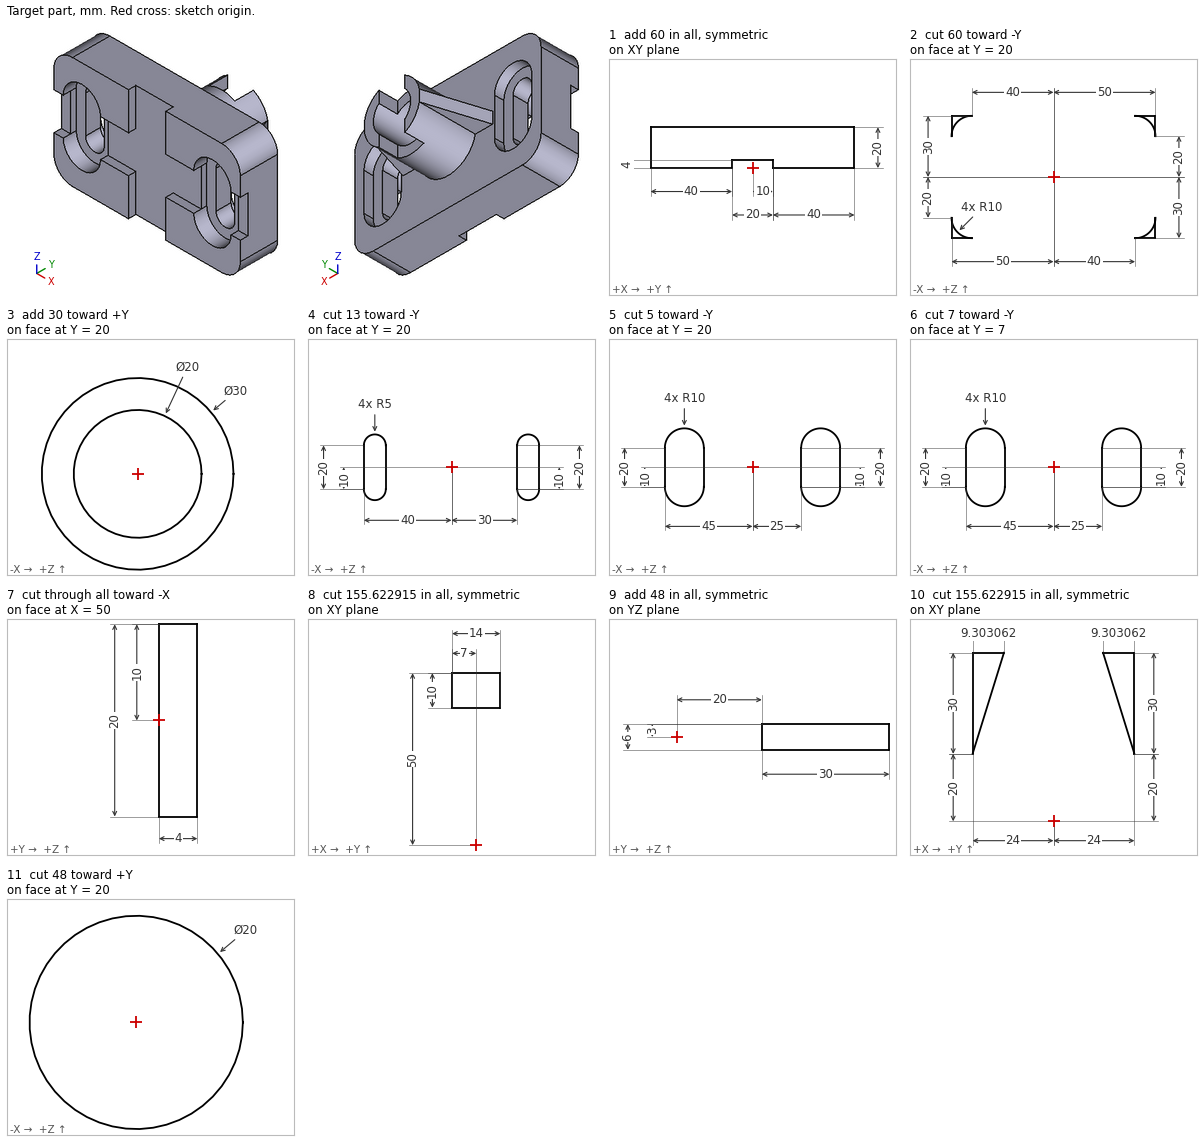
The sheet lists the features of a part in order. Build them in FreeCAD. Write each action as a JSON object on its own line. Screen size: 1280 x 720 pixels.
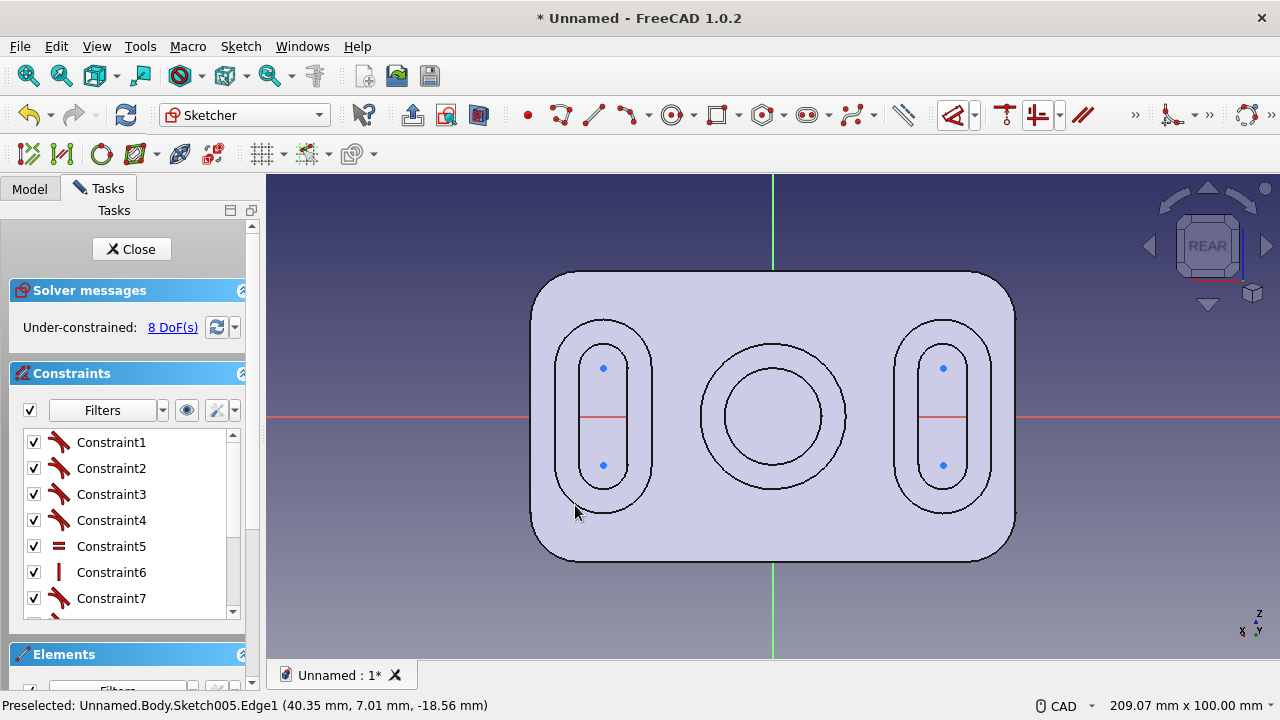
{"action": "left_click", "coordinate": [915, 505]}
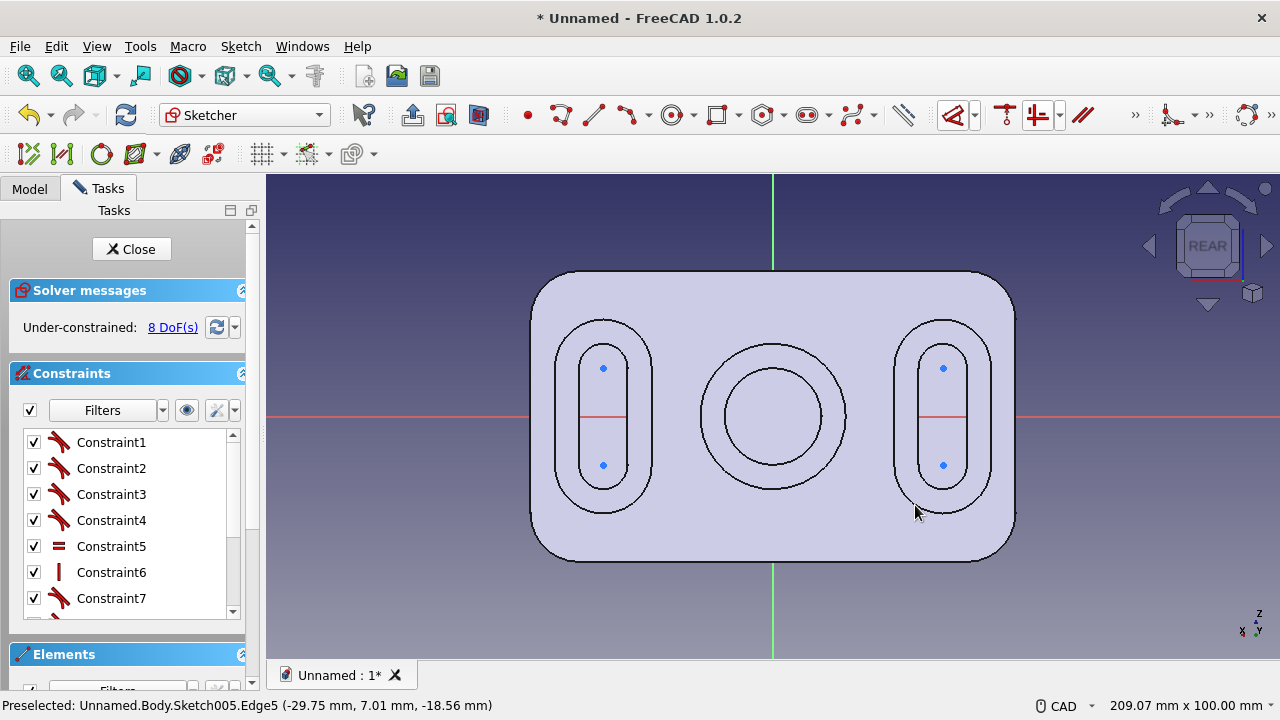
{"action": "key", "text": "e"}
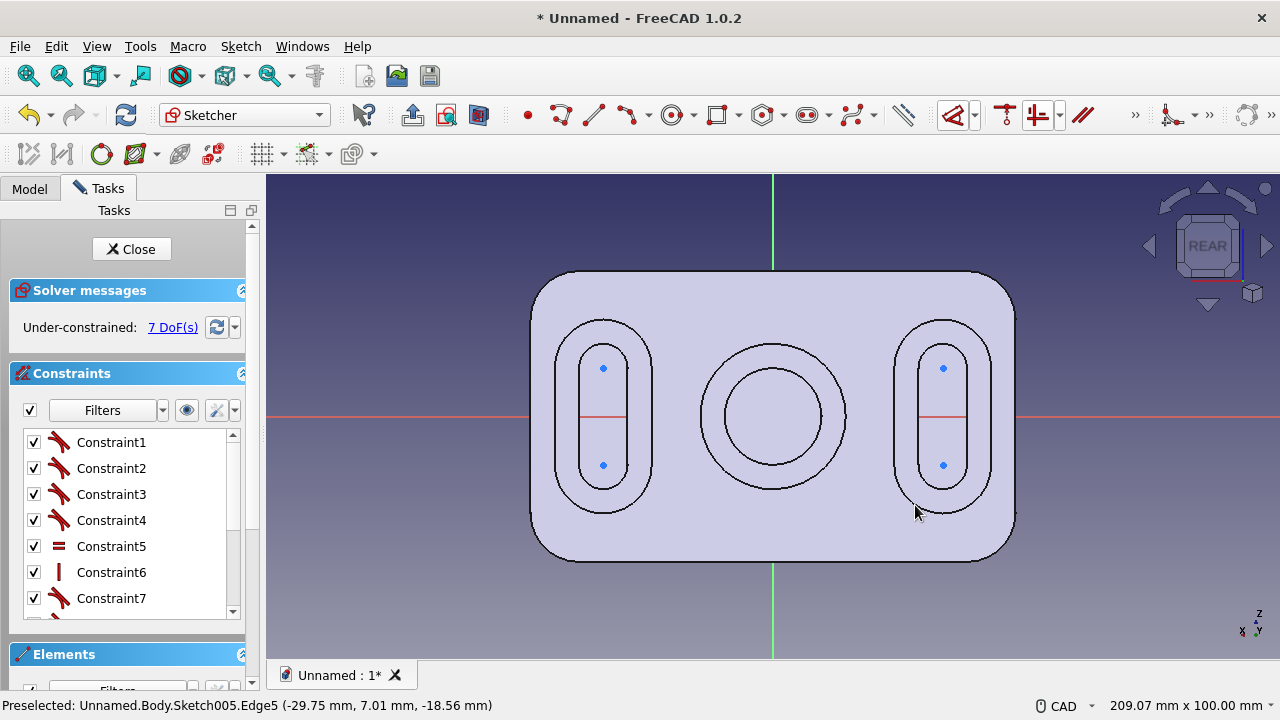
{"action": "left_click", "coordinate": [575, 505]}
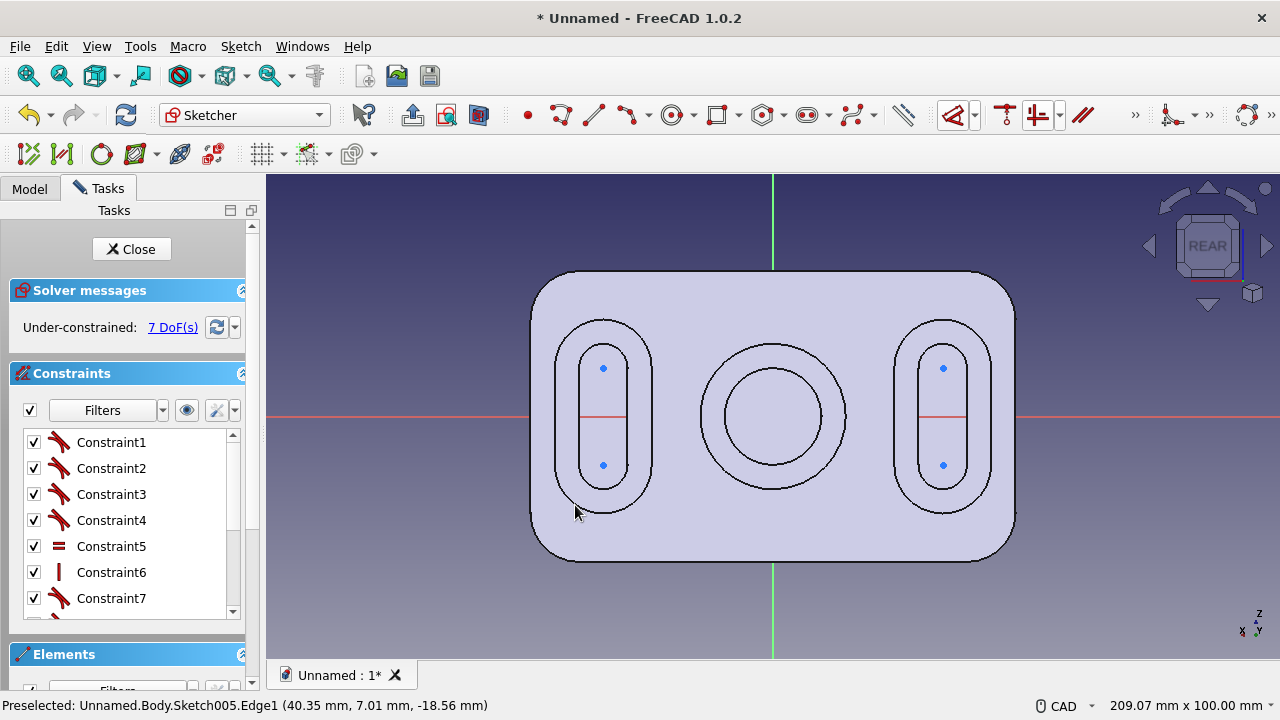
{"action": "left_click", "coordinate": [974, 116]}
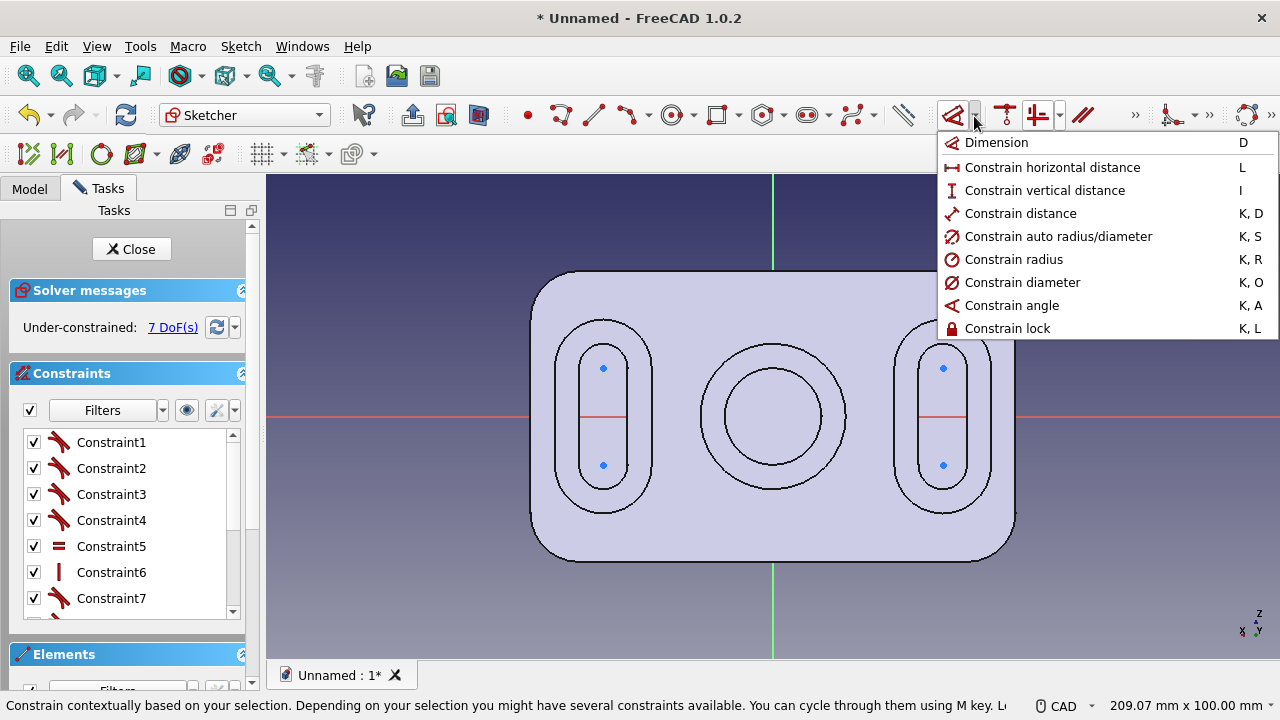
{"action": "left_click", "coordinate": [1108, 260]}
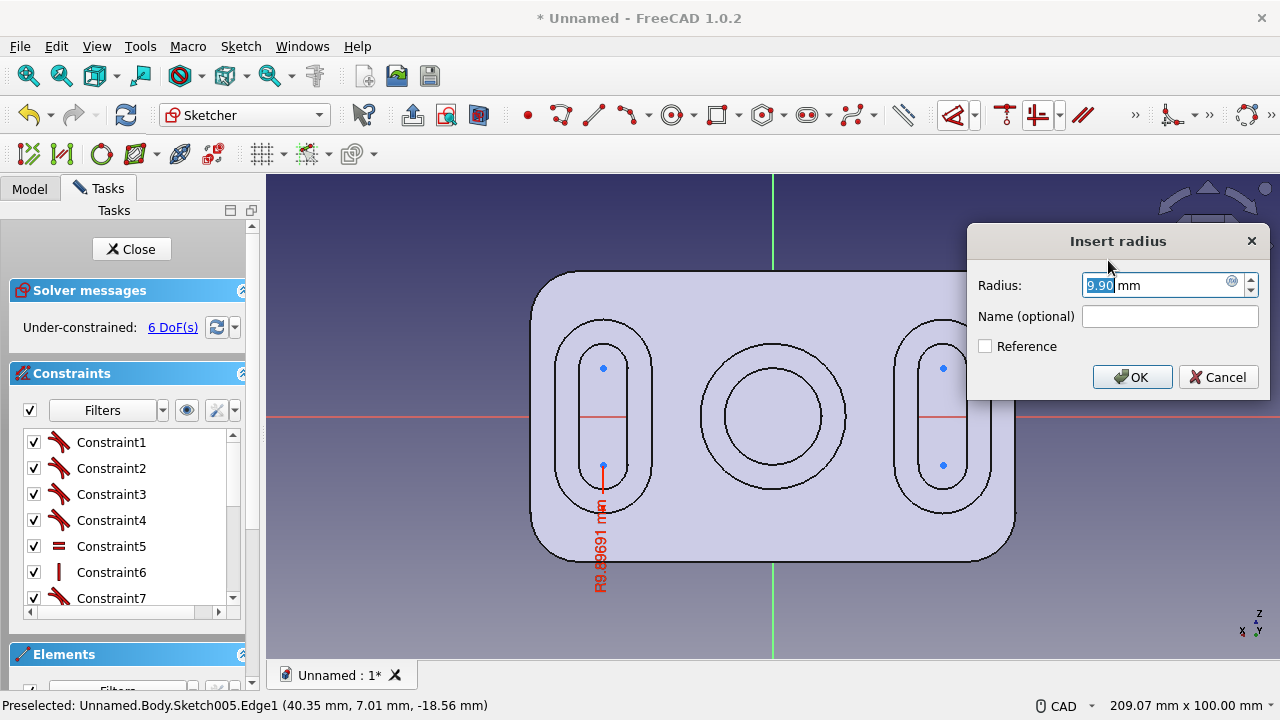
{"action": "type", "text": "10"}
{"action": "key", "text": "Return"}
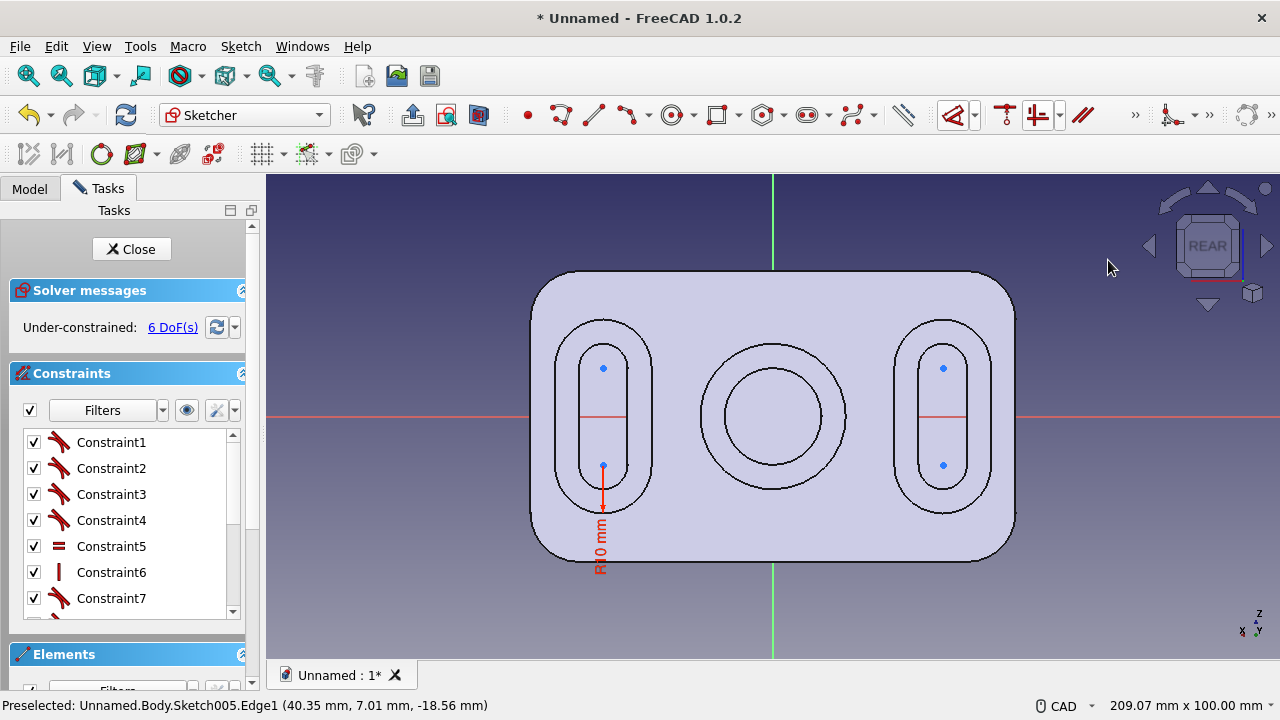
{"action": "left_click", "coordinate": [555, 437]}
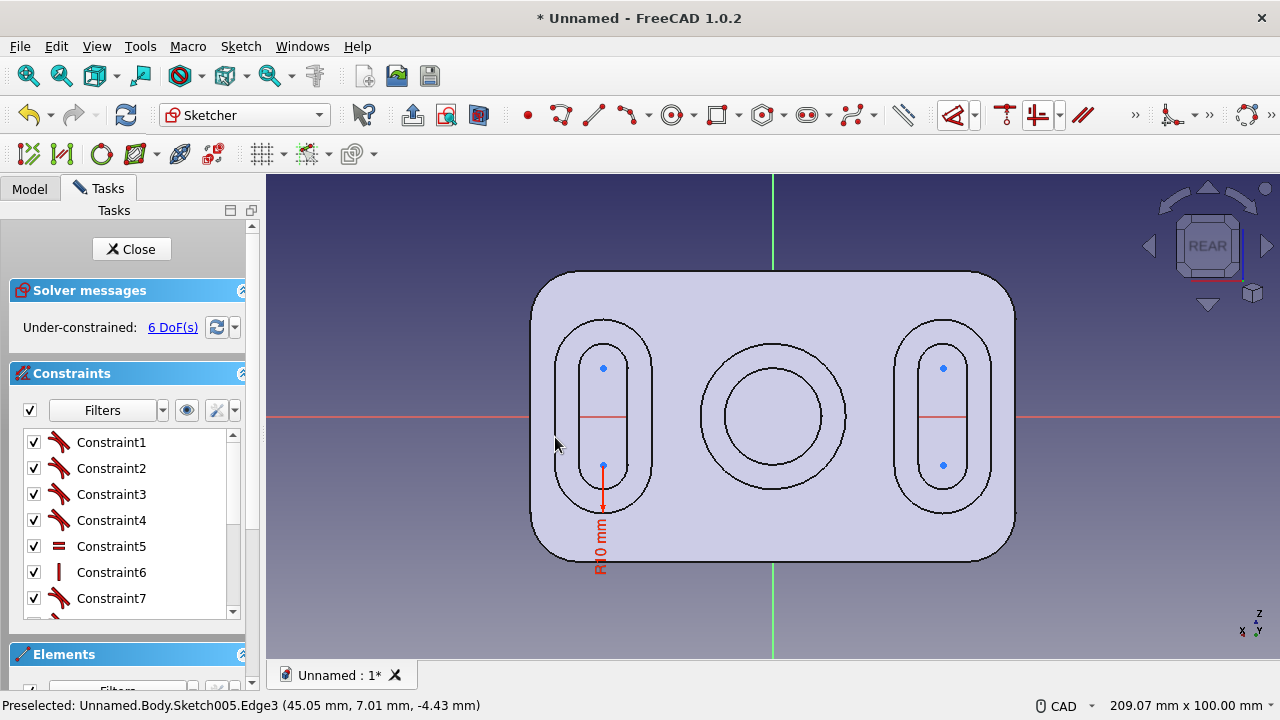
{"action": "key", "text": "i"}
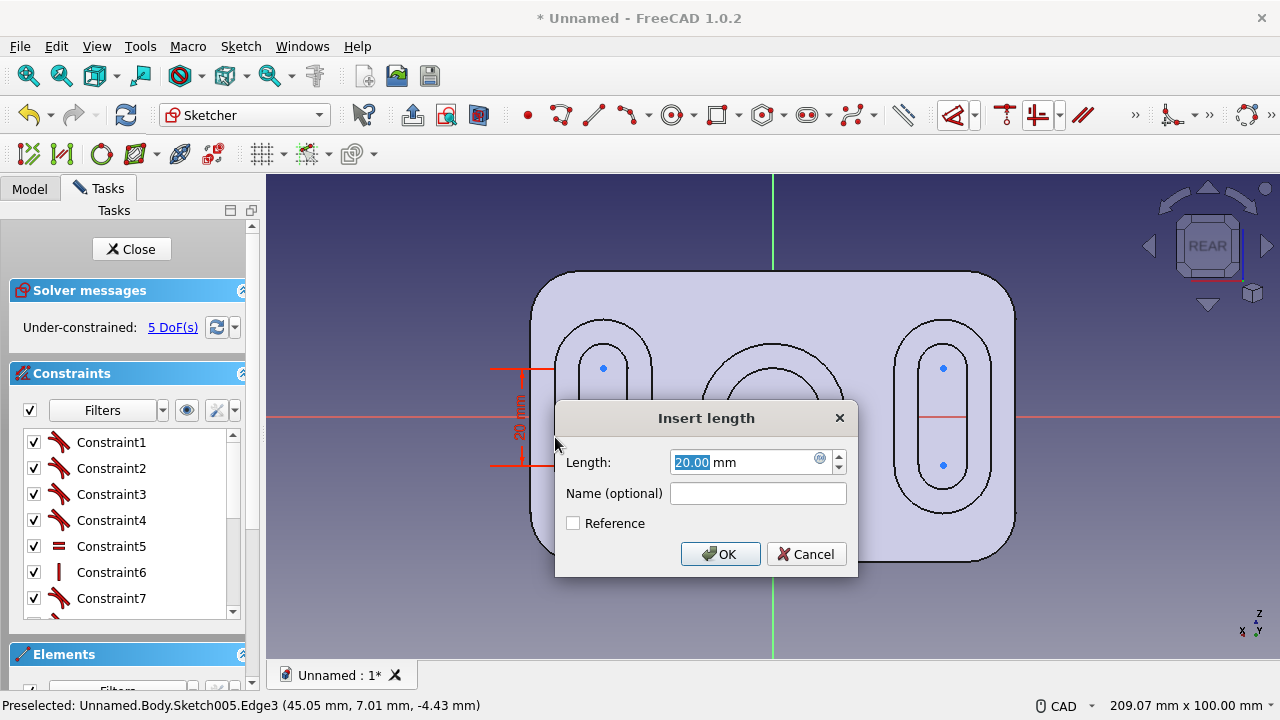
{"action": "type", "text": "20"}
{"action": "key", "text": "Return"}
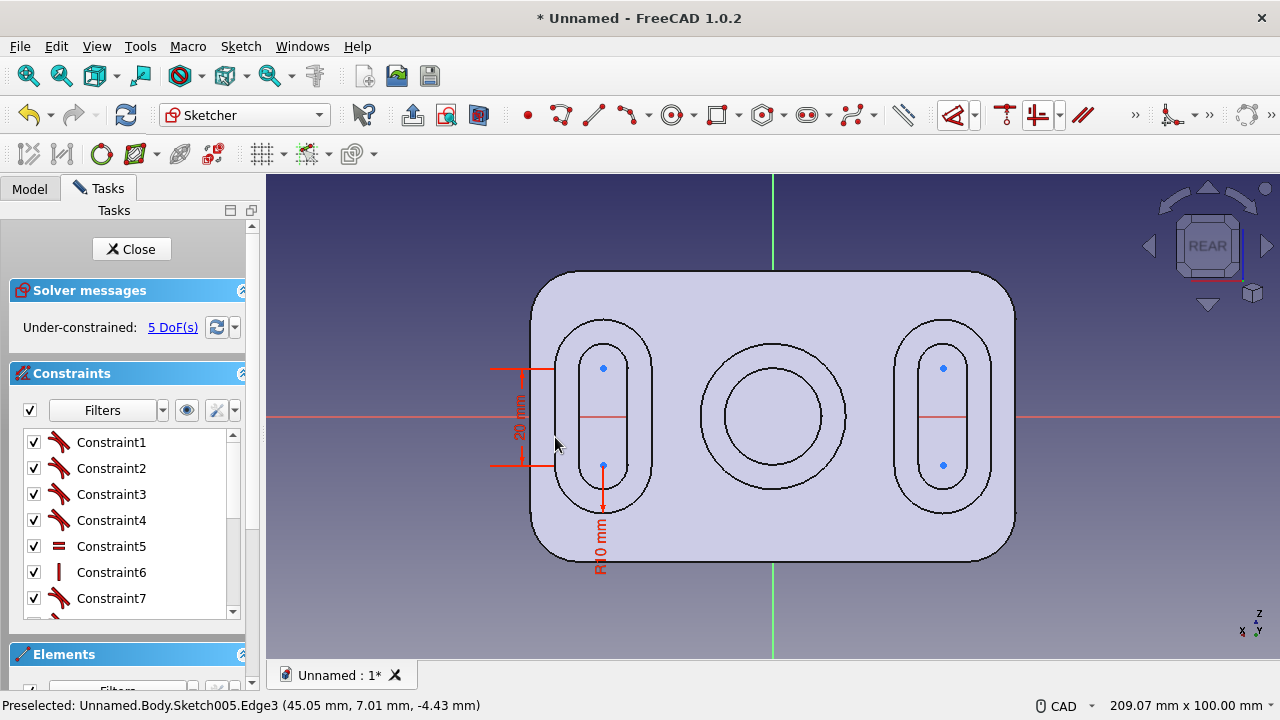
{"action": "left_click", "coordinate": [894, 437]}